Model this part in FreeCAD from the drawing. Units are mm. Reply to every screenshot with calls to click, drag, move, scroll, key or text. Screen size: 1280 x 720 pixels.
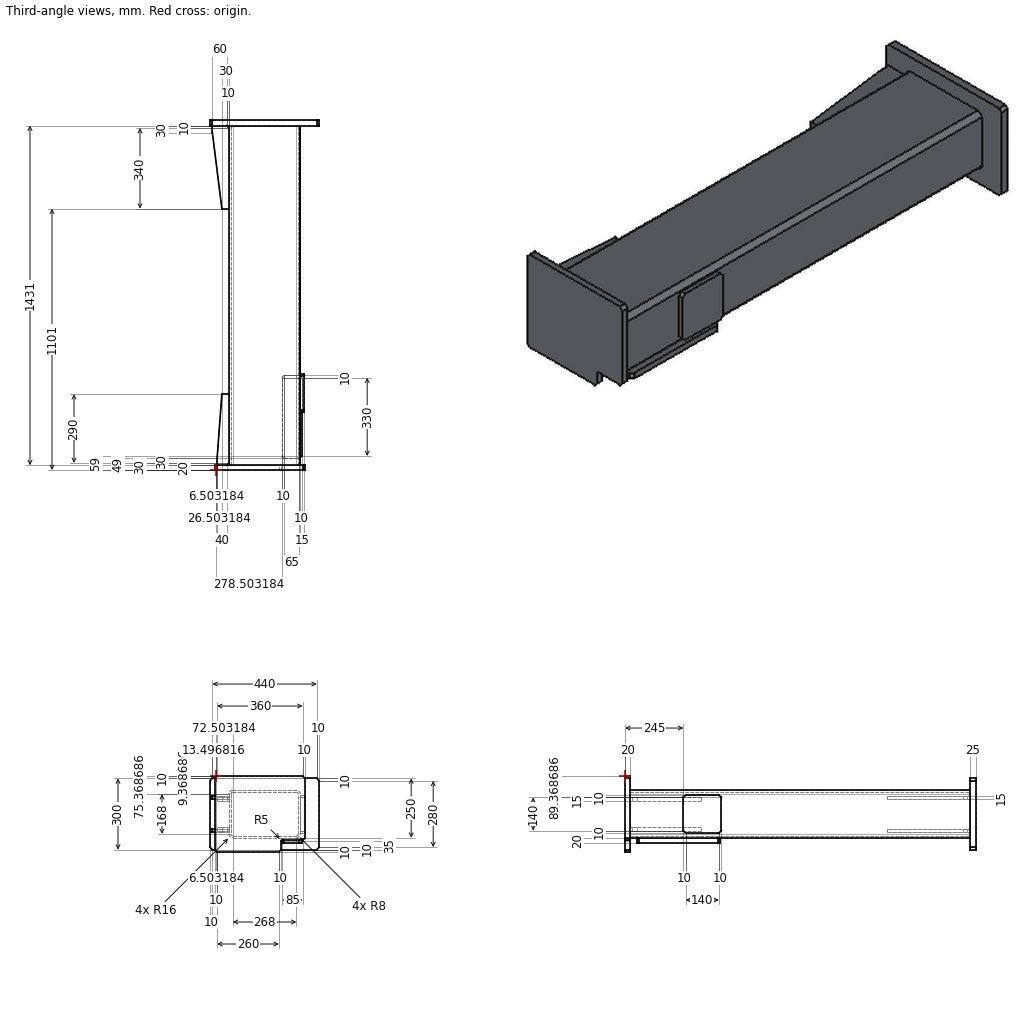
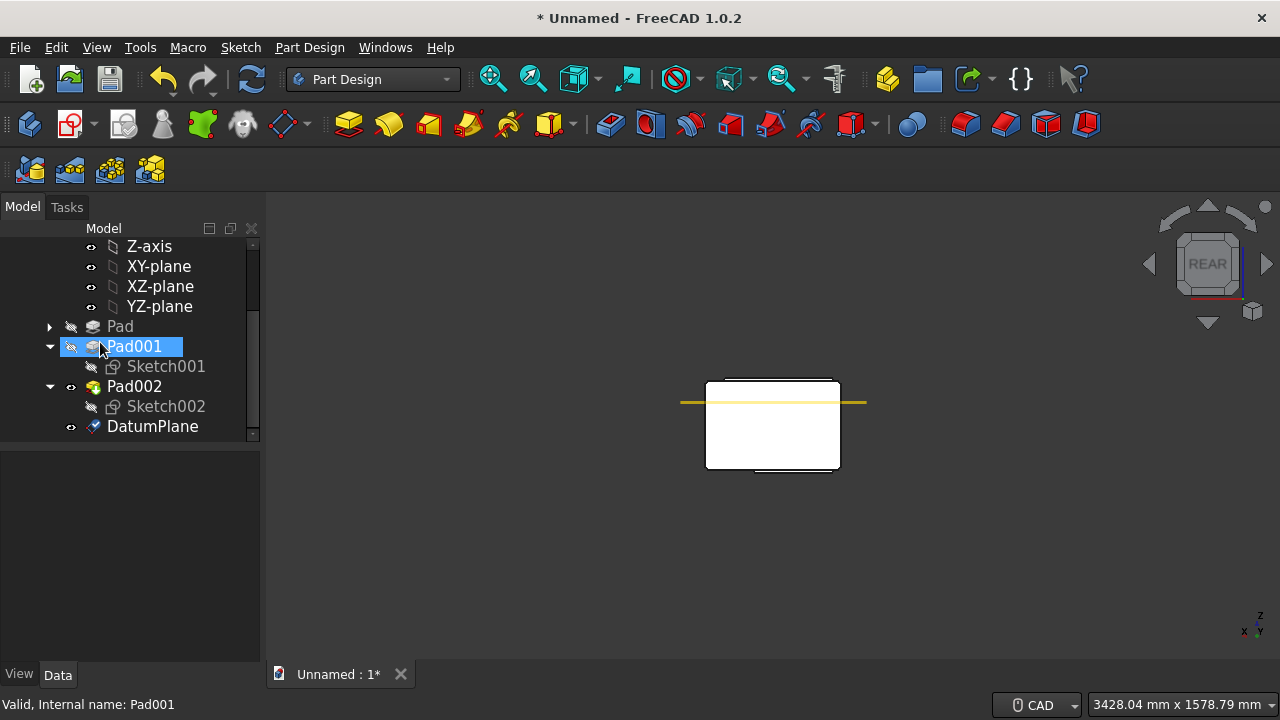
click(116, 427)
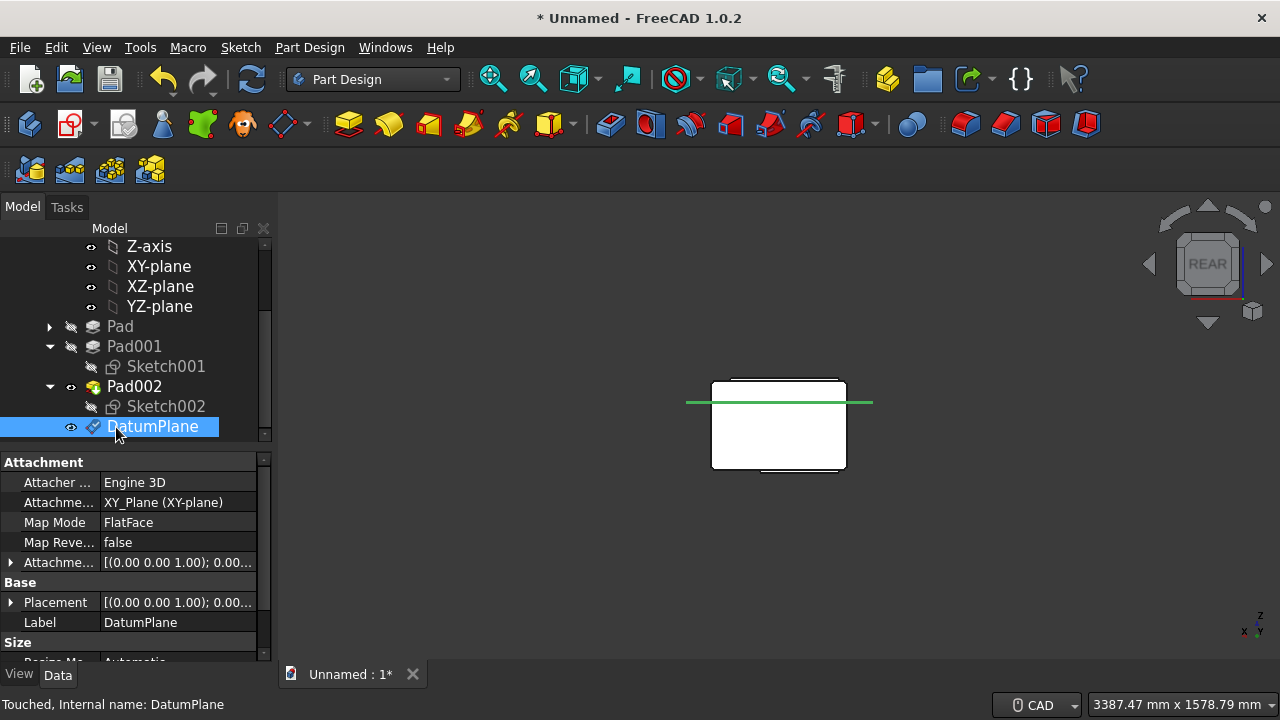
click(70, 124)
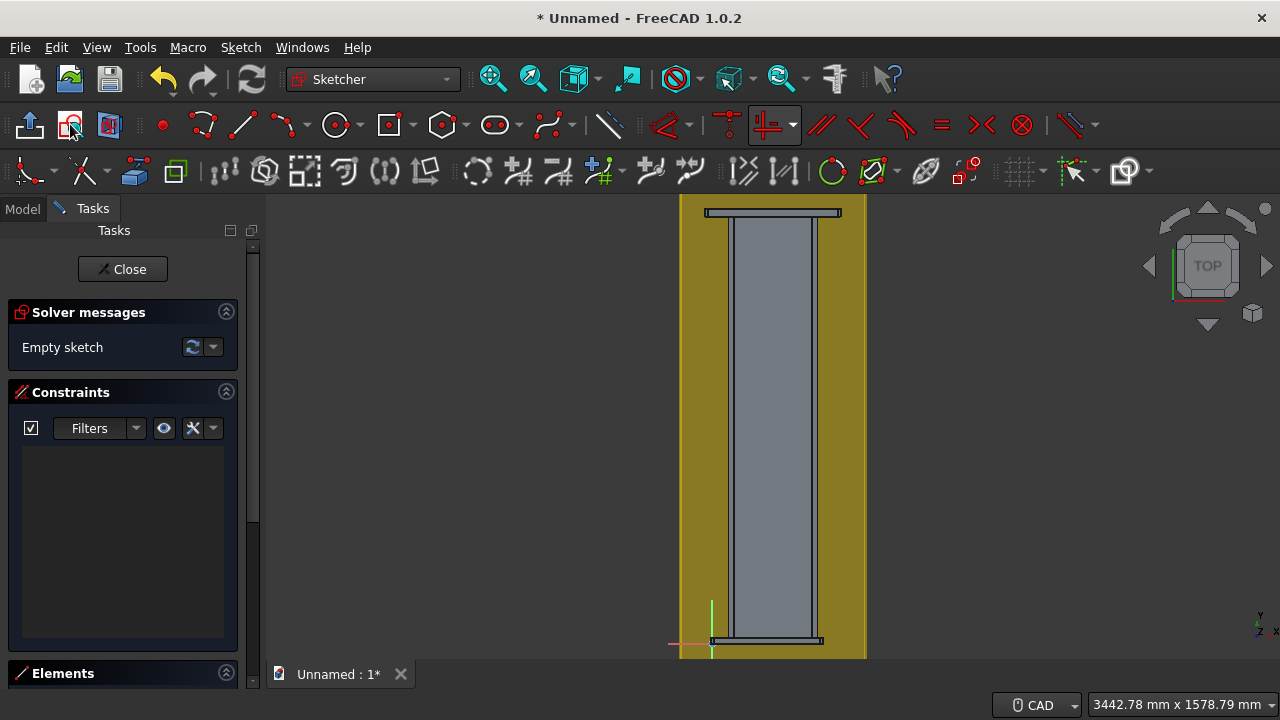
click(110, 126)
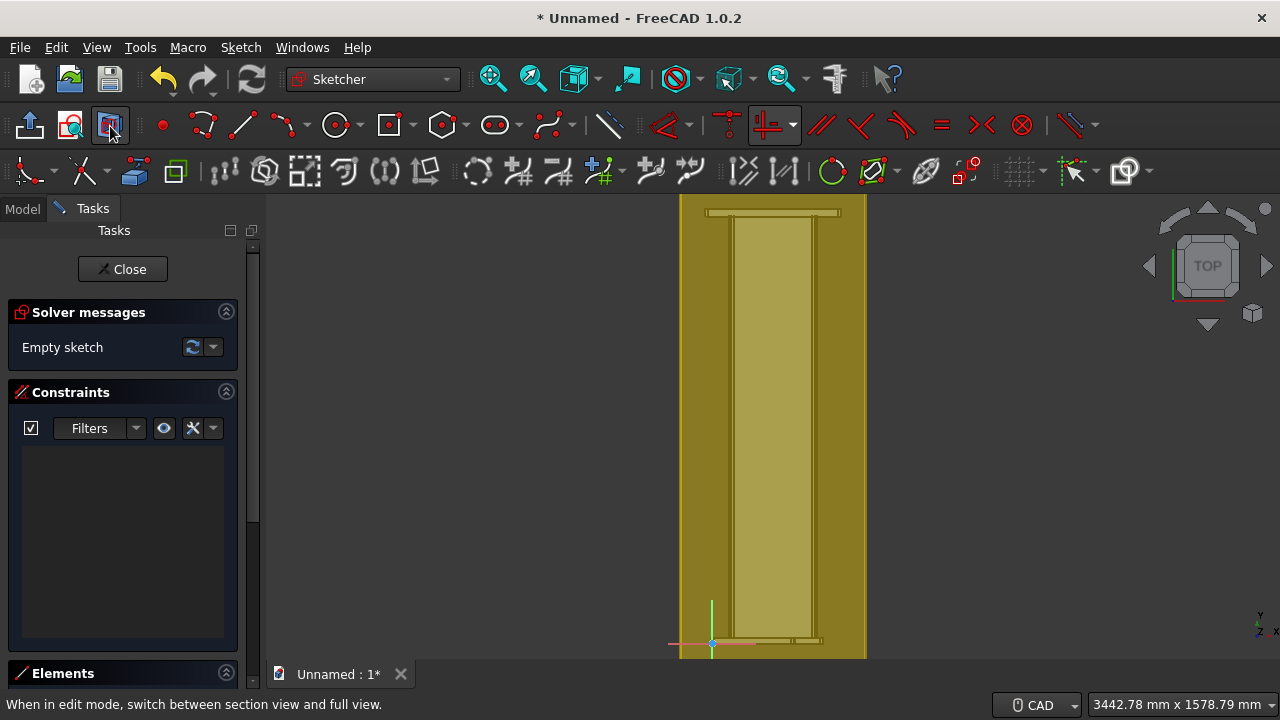
scroll(704, 426, down, 5)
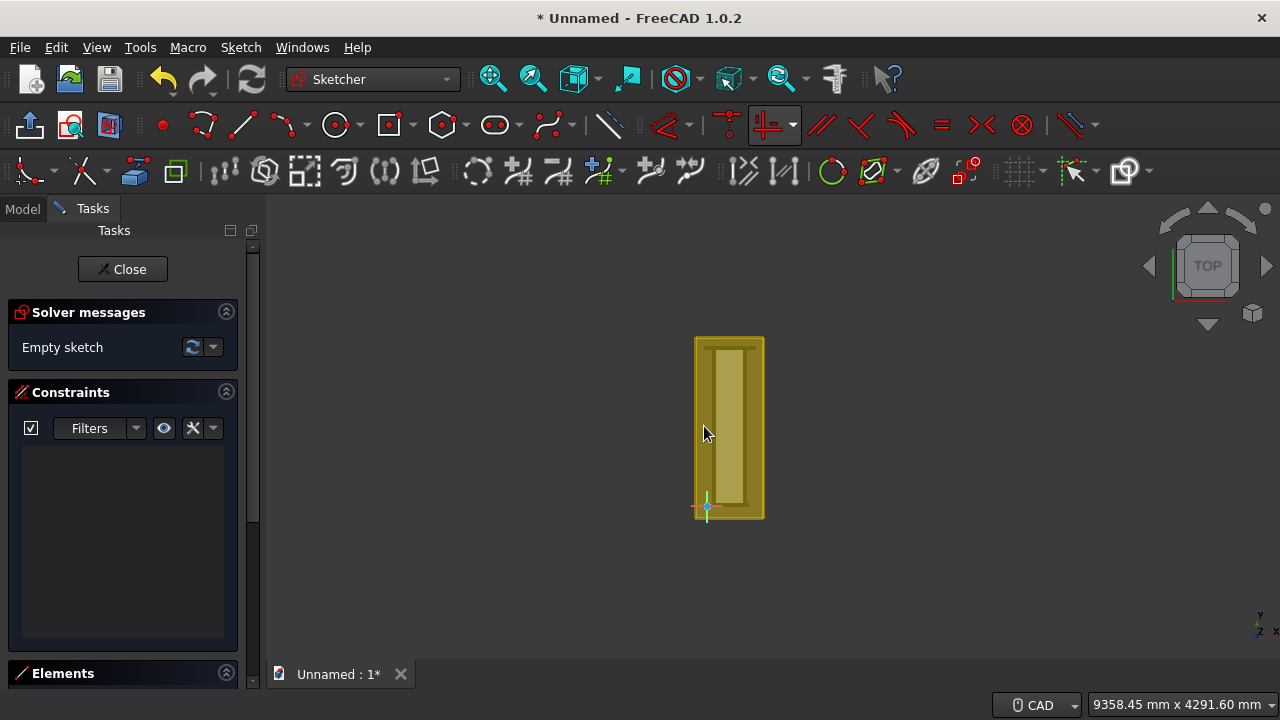
scroll(710, 359, up, 10)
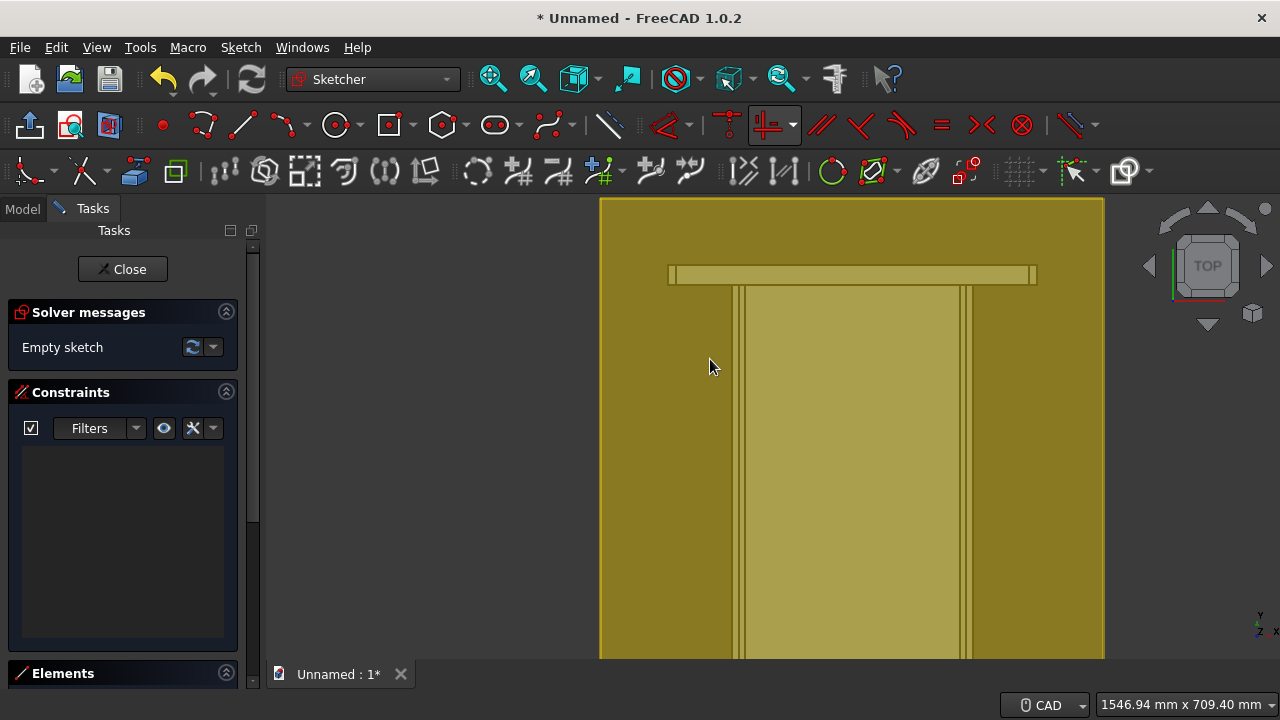
click(204, 126)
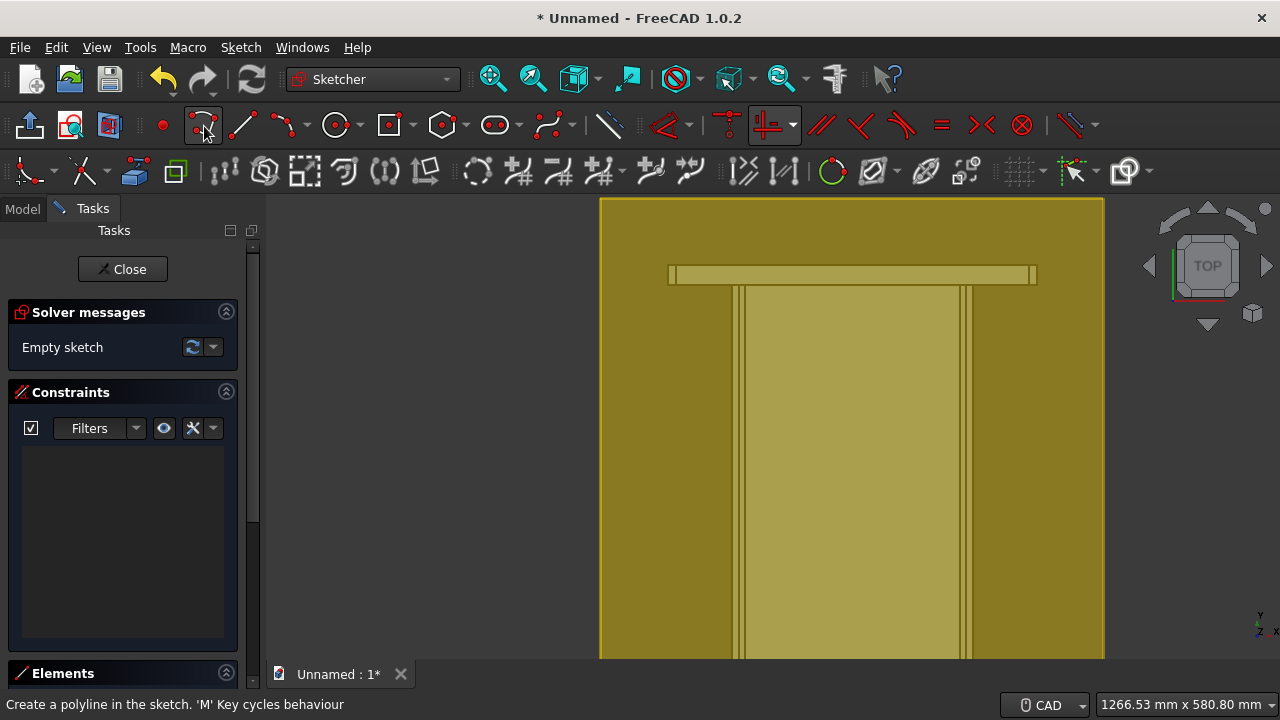
click(708, 565)
click(732, 565)
click(732, 293)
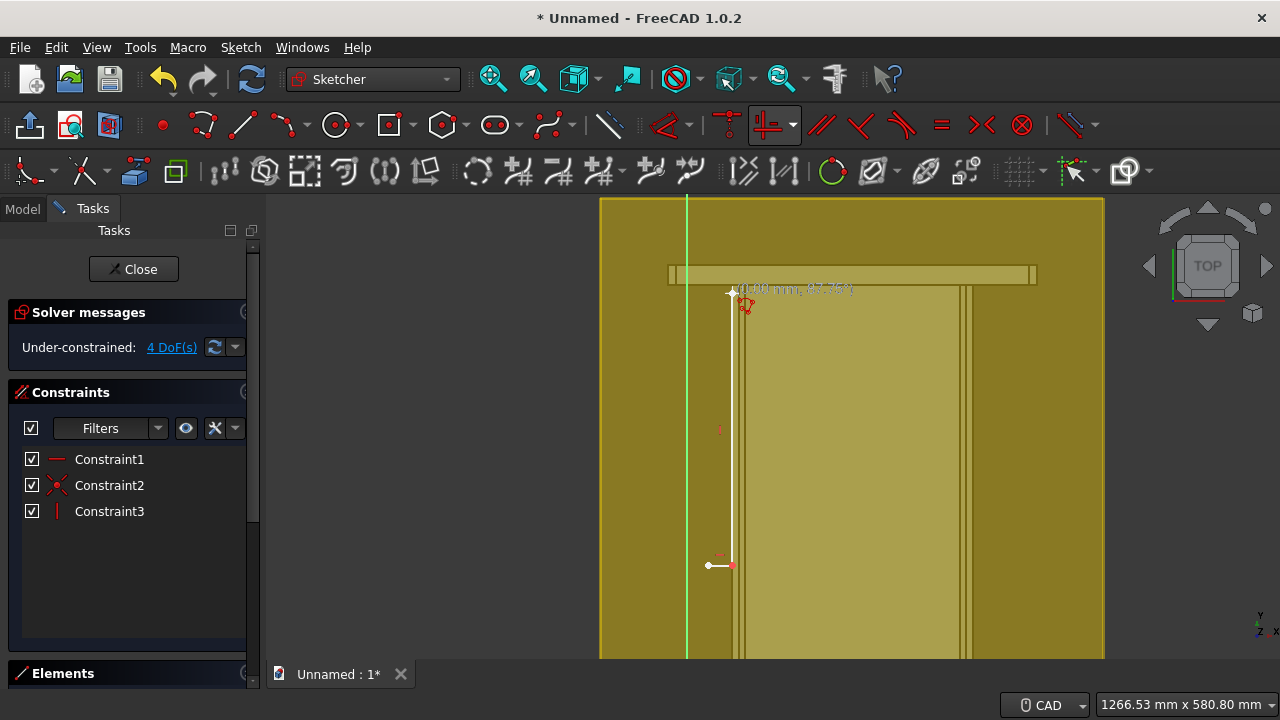
scroll(724, 285, up, 2)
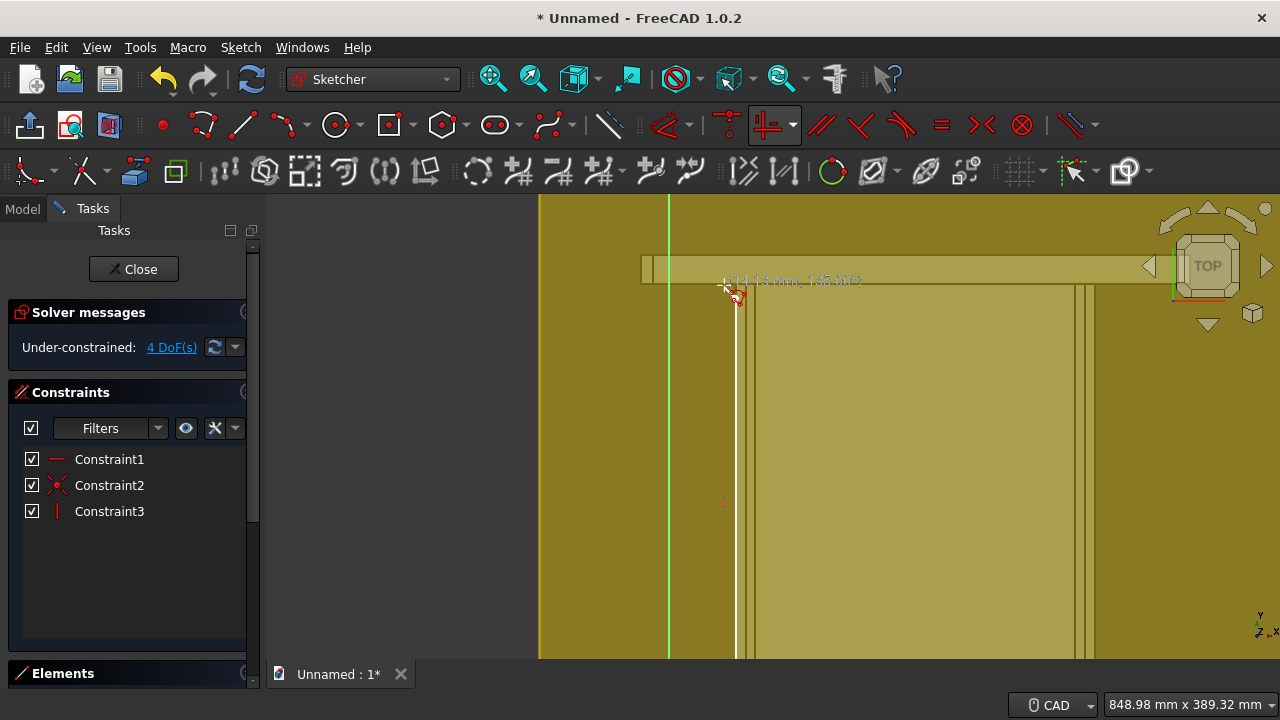
click(724, 284)
click(653, 284)
click(653, 320)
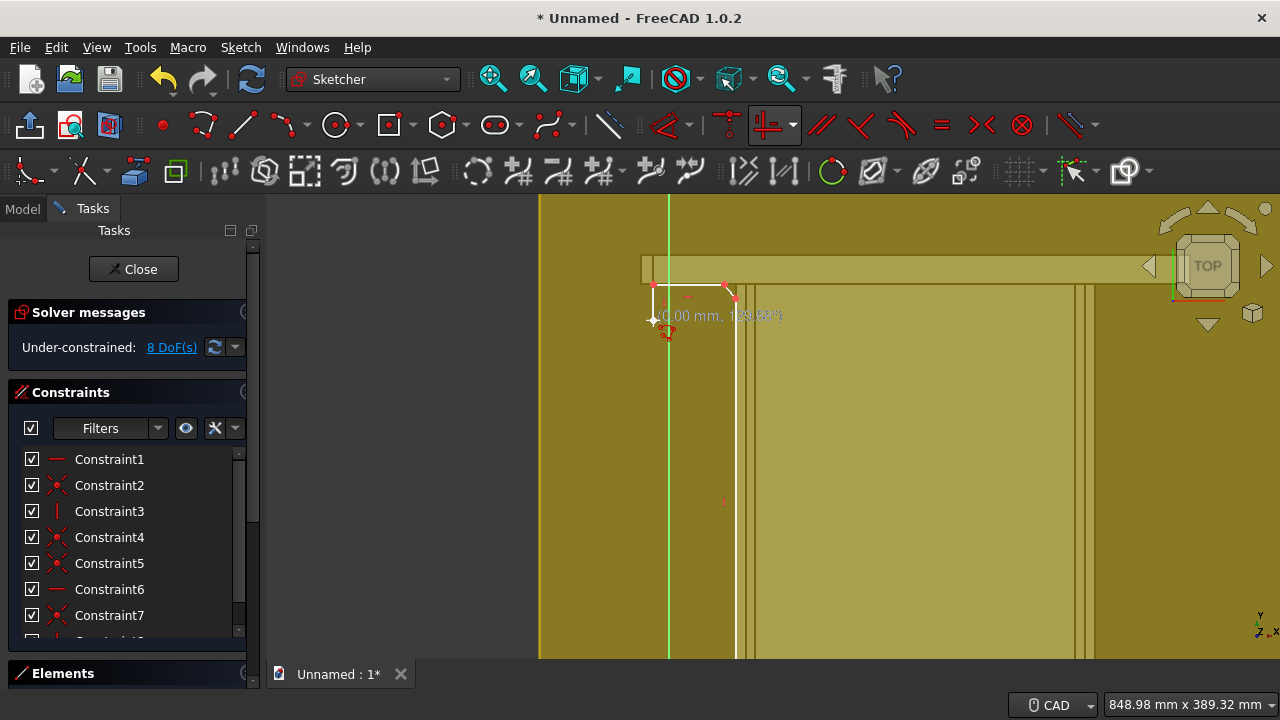
scroll(725, 290, down, 2)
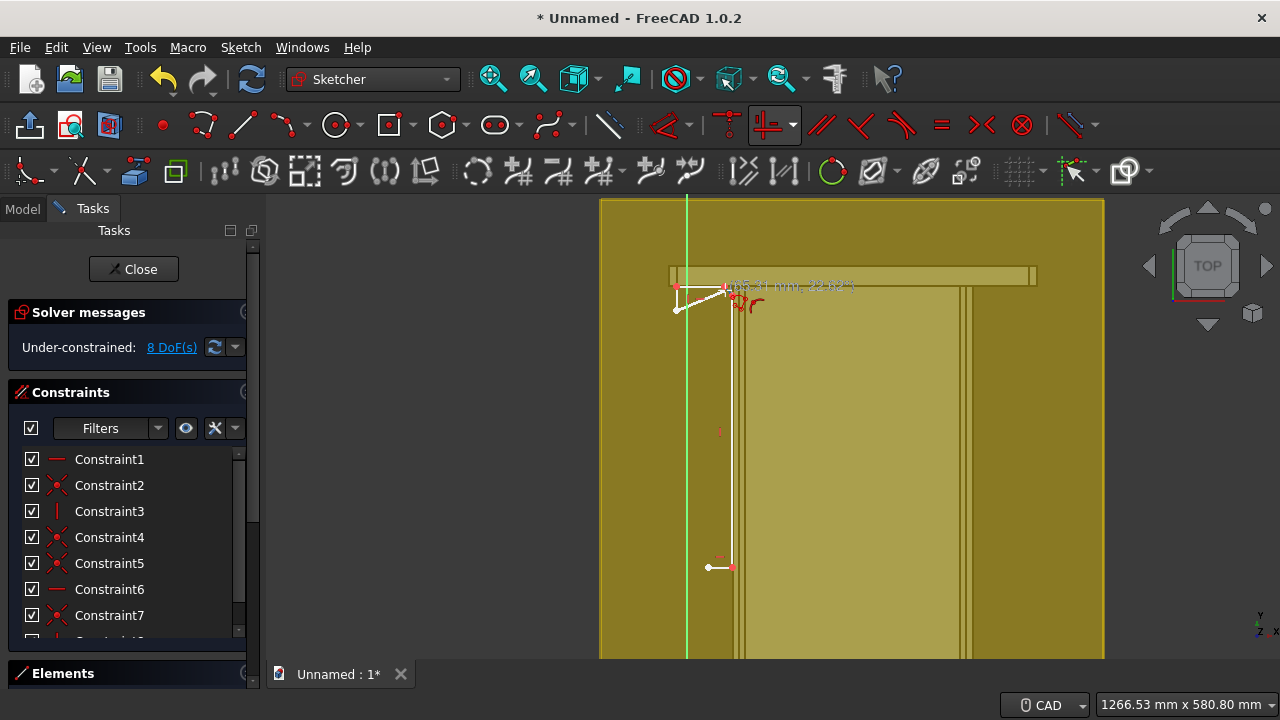
scroll(709, 567, up, 2)